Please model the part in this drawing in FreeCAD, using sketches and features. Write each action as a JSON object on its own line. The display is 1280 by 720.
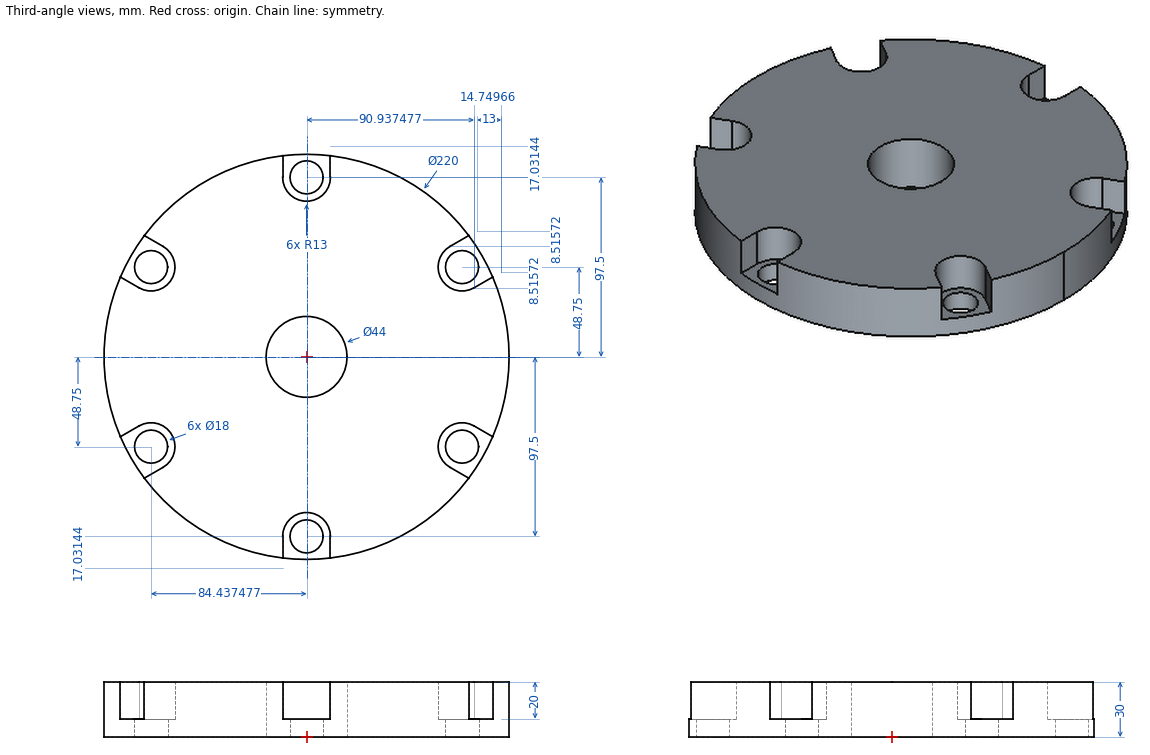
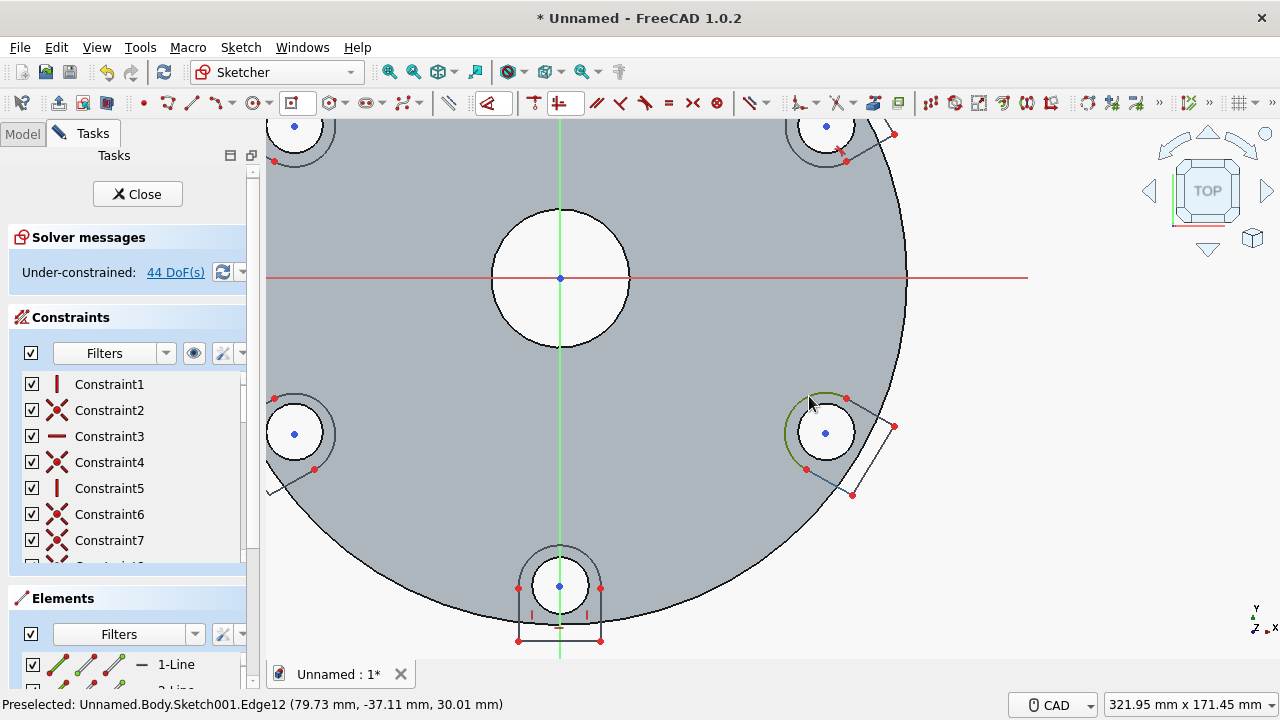
{"action": "left_click", "coordinate": [646, 104]}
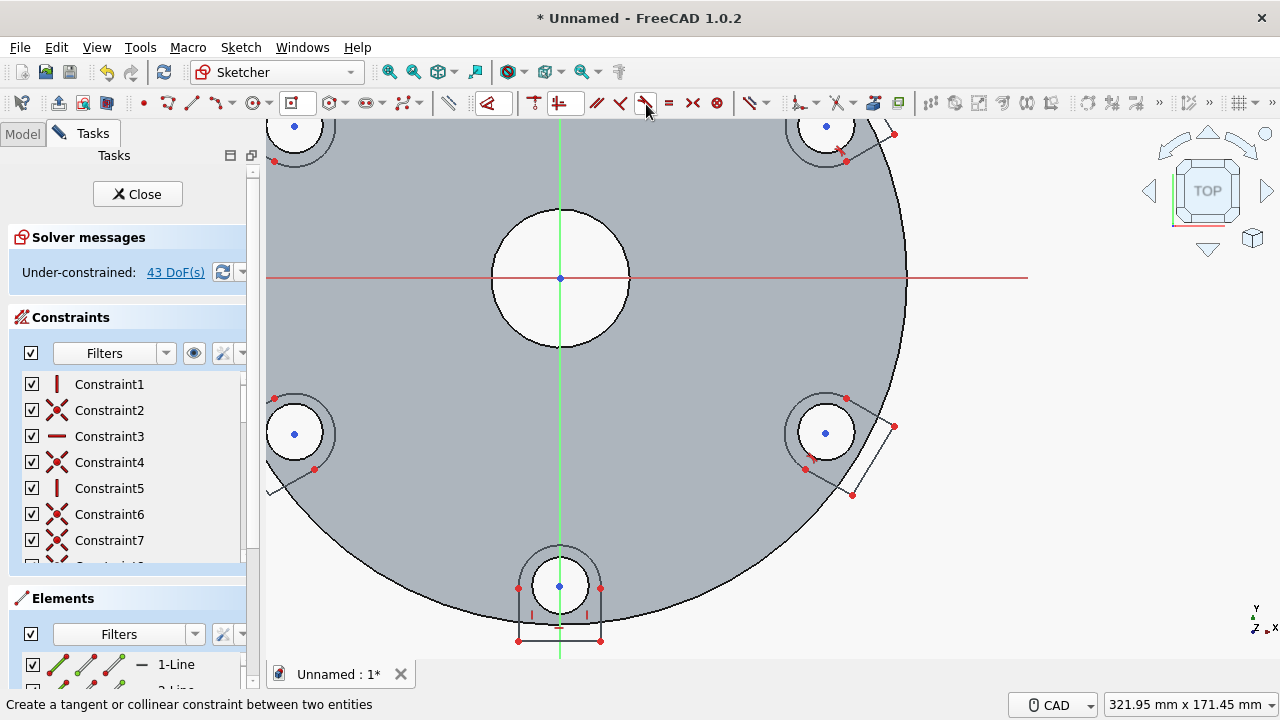
{"action": "left_click", "coordinate": [880, 418]}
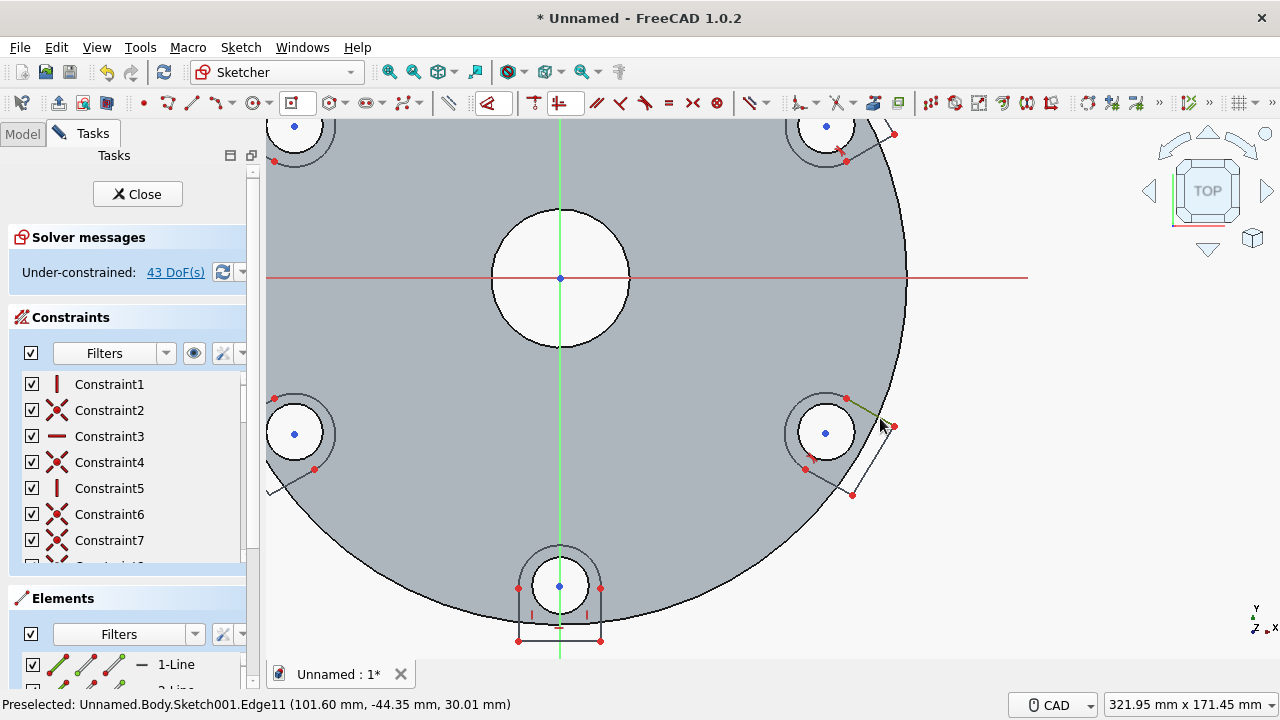
{"action": "left_click", "coordinate": [809, 396]}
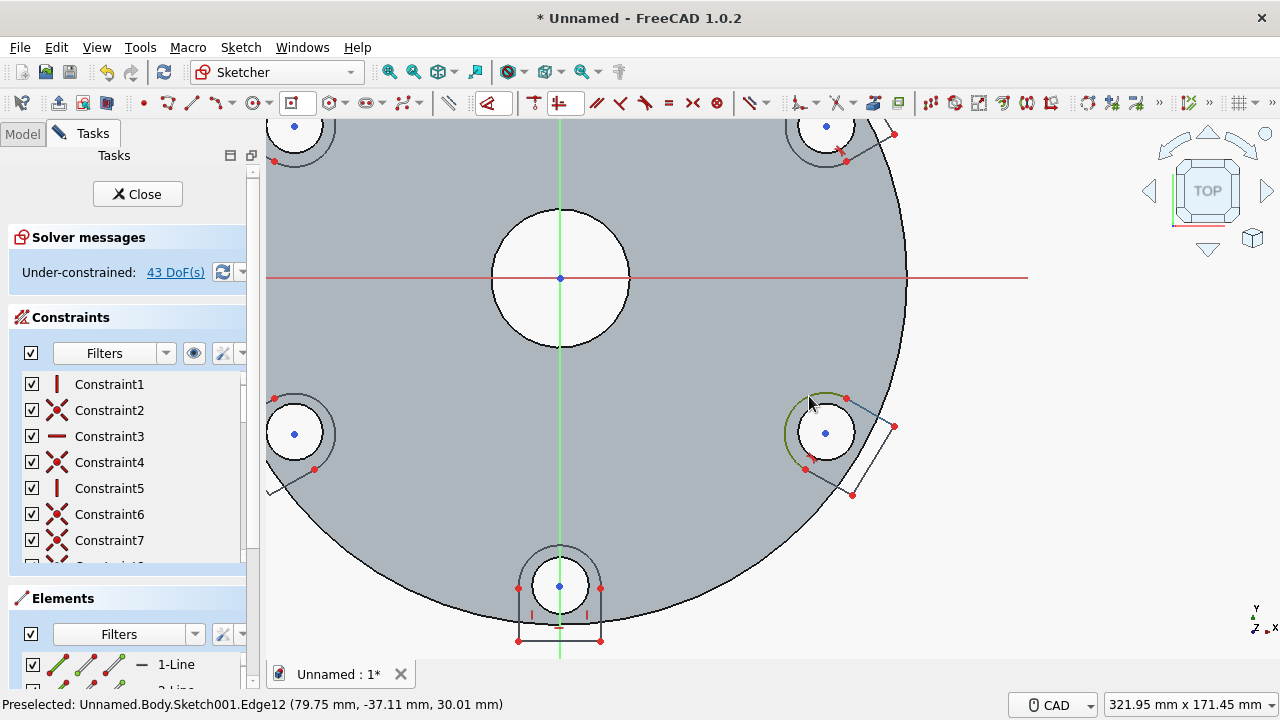
{"action": "left_click", "coordinate": [646, 104]}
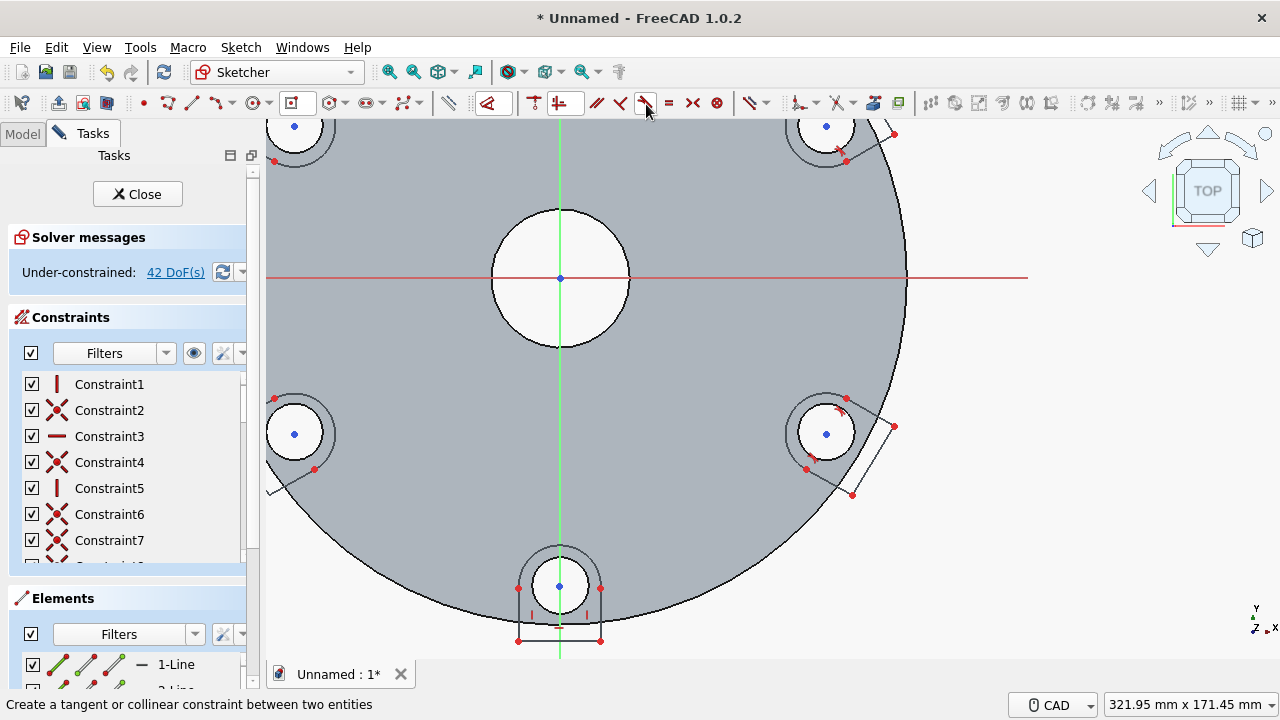
{"action": "left_click", "coordinate": [519, 604]}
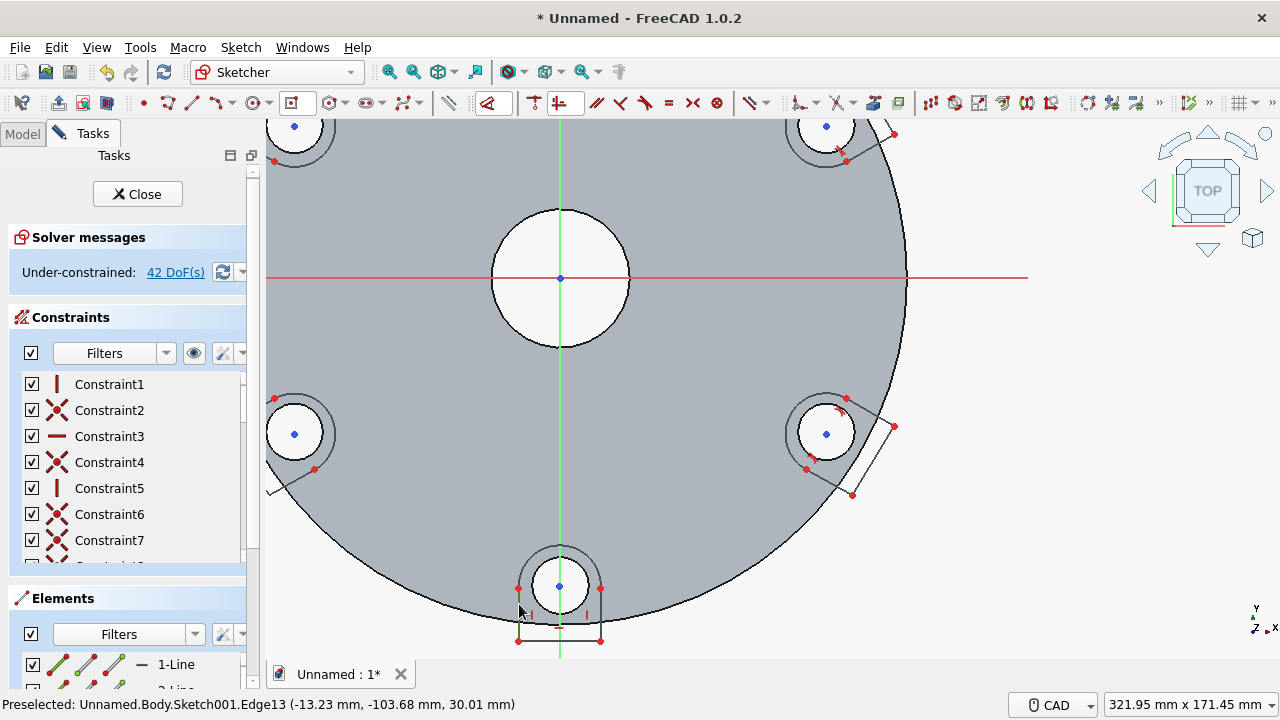
{"action": "left_click", "coordinate": [585, 554]}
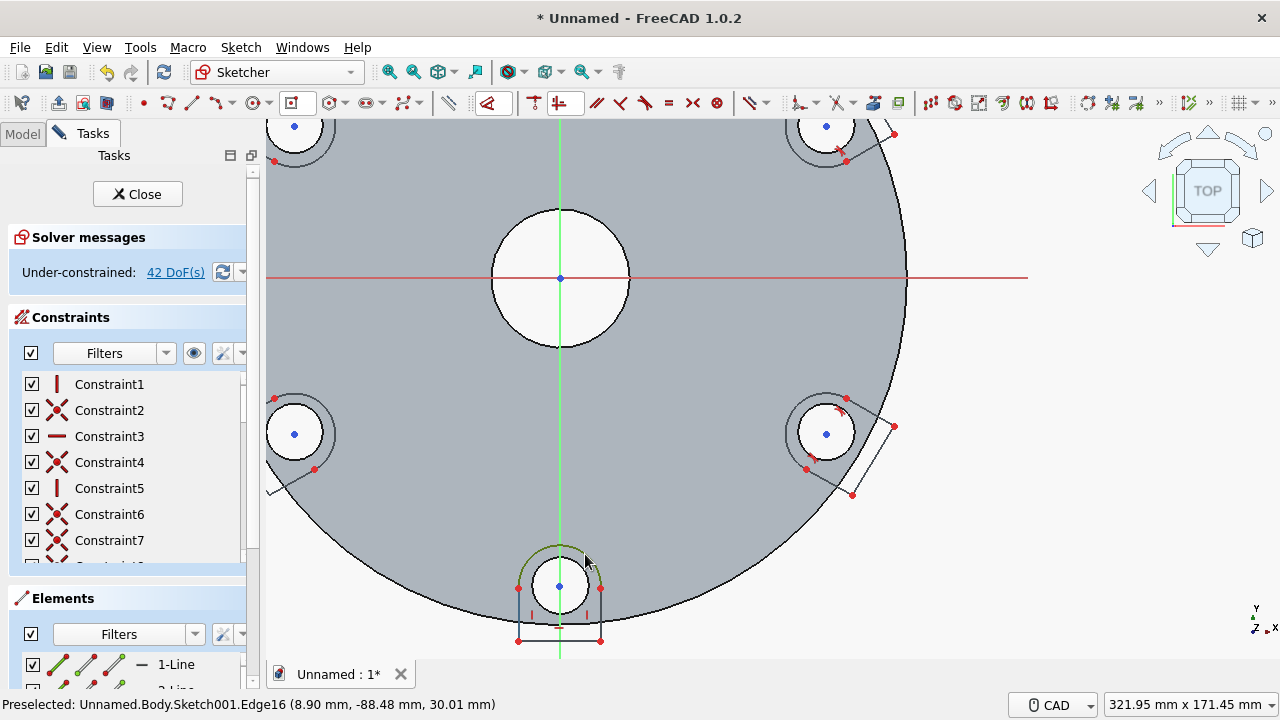
{"action": "left_click", "coordinate": [646, 104]}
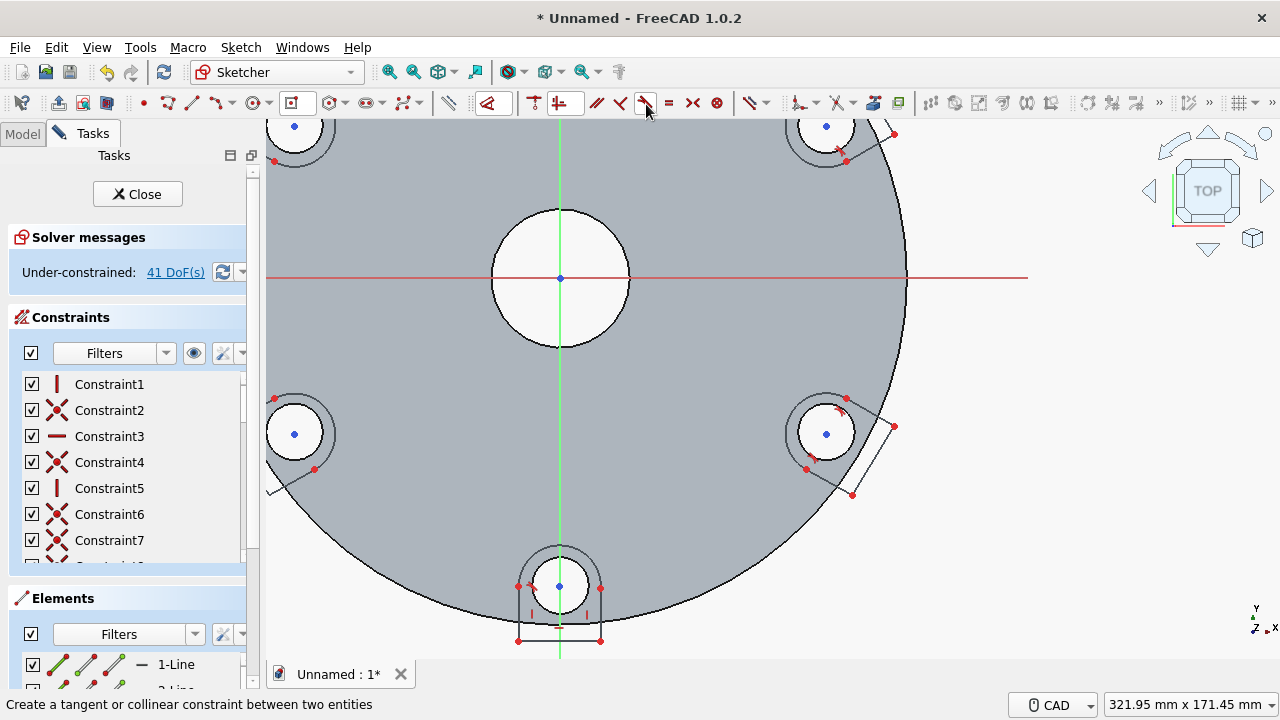
{"action": "left_click", "coordinate": [601, 625]}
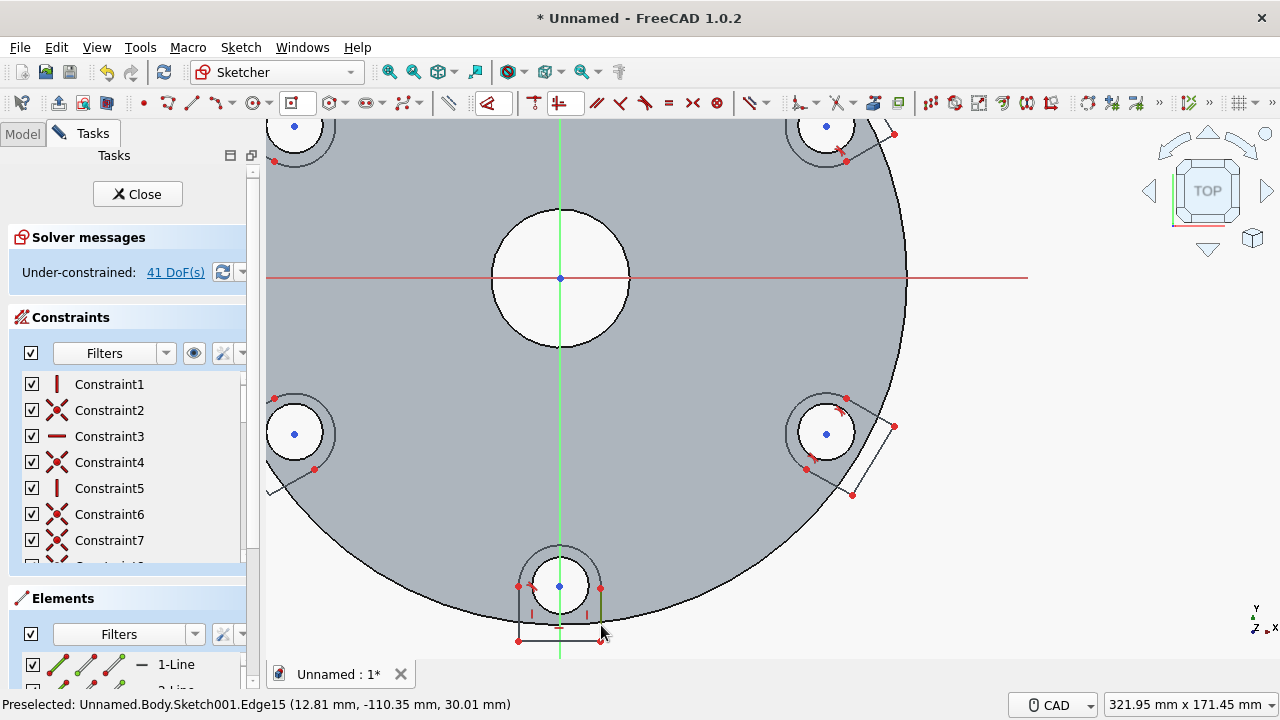
{"action": "left_click", "coordinate": [585, 554]}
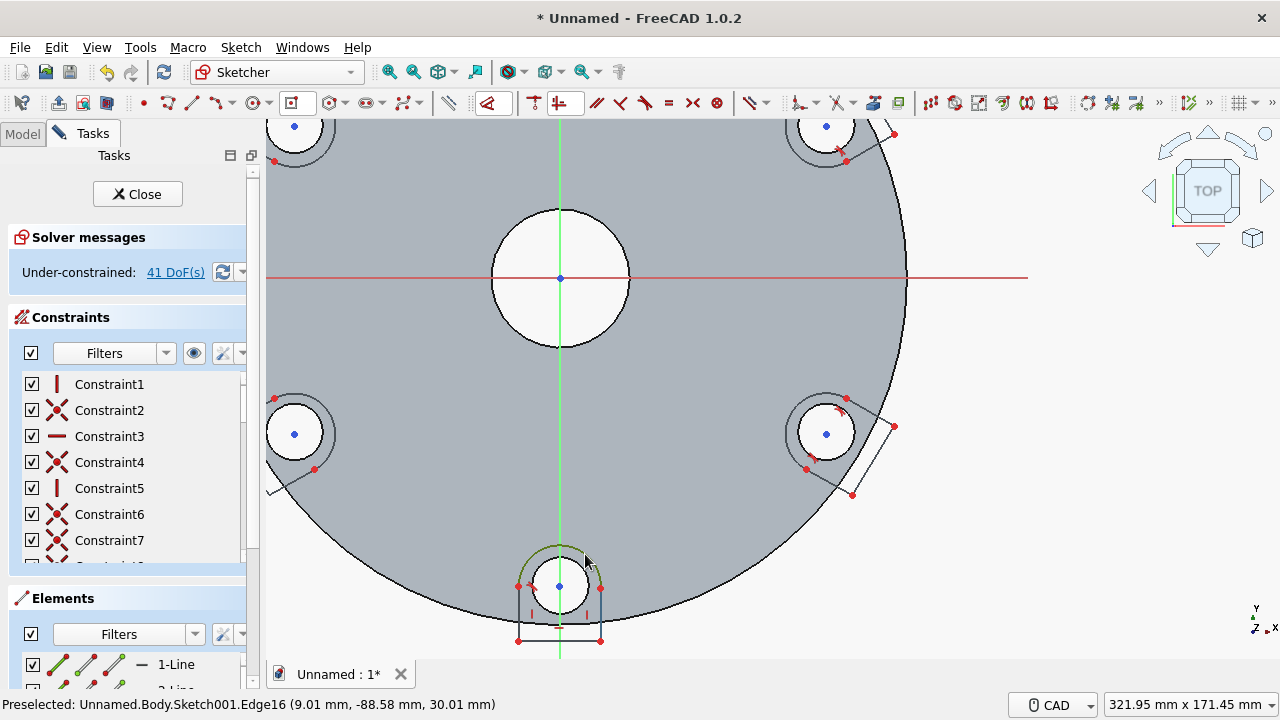
{"action": "left_click", "coordinate": [646, 104]}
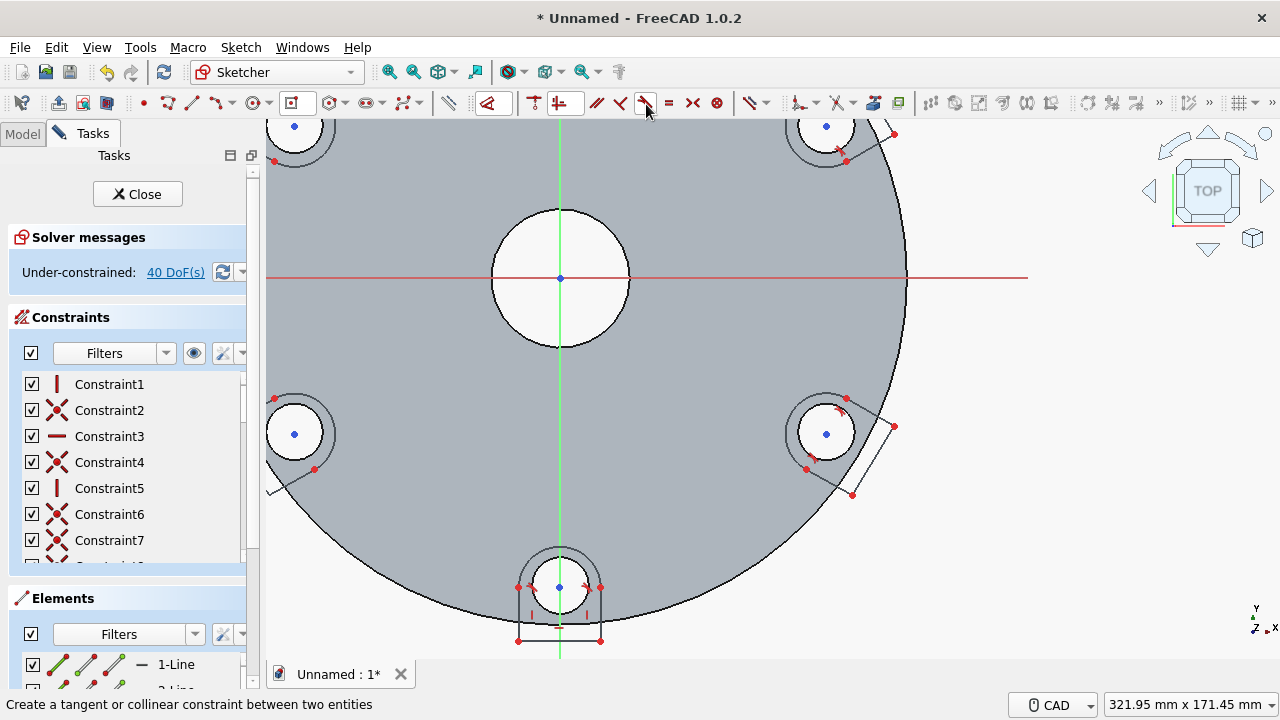
{"action": "scroll", "coordinate": [822, 479], "scroll_direction": "down", "scroll_amount": 4}